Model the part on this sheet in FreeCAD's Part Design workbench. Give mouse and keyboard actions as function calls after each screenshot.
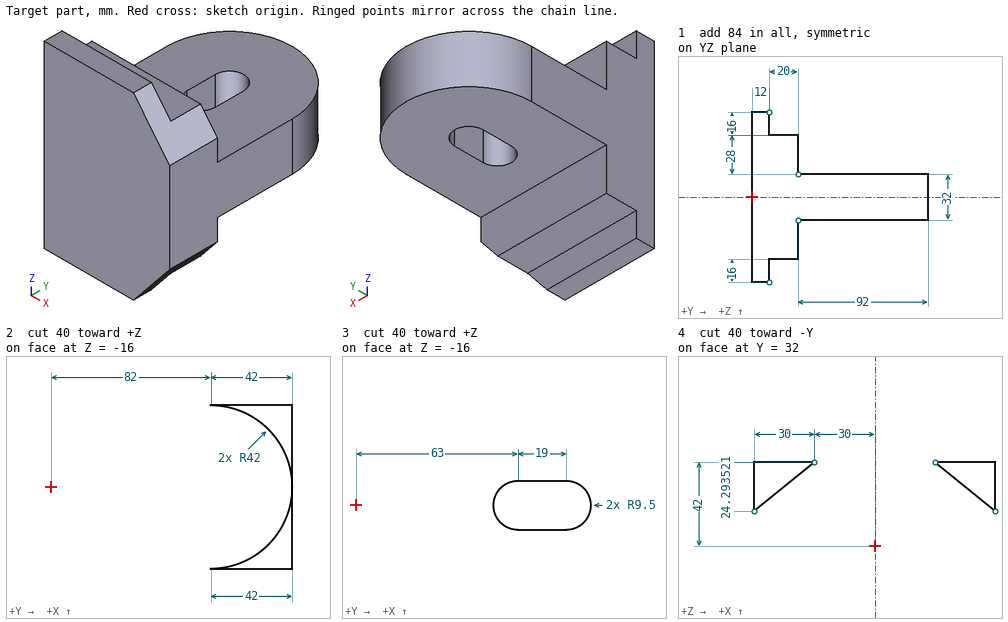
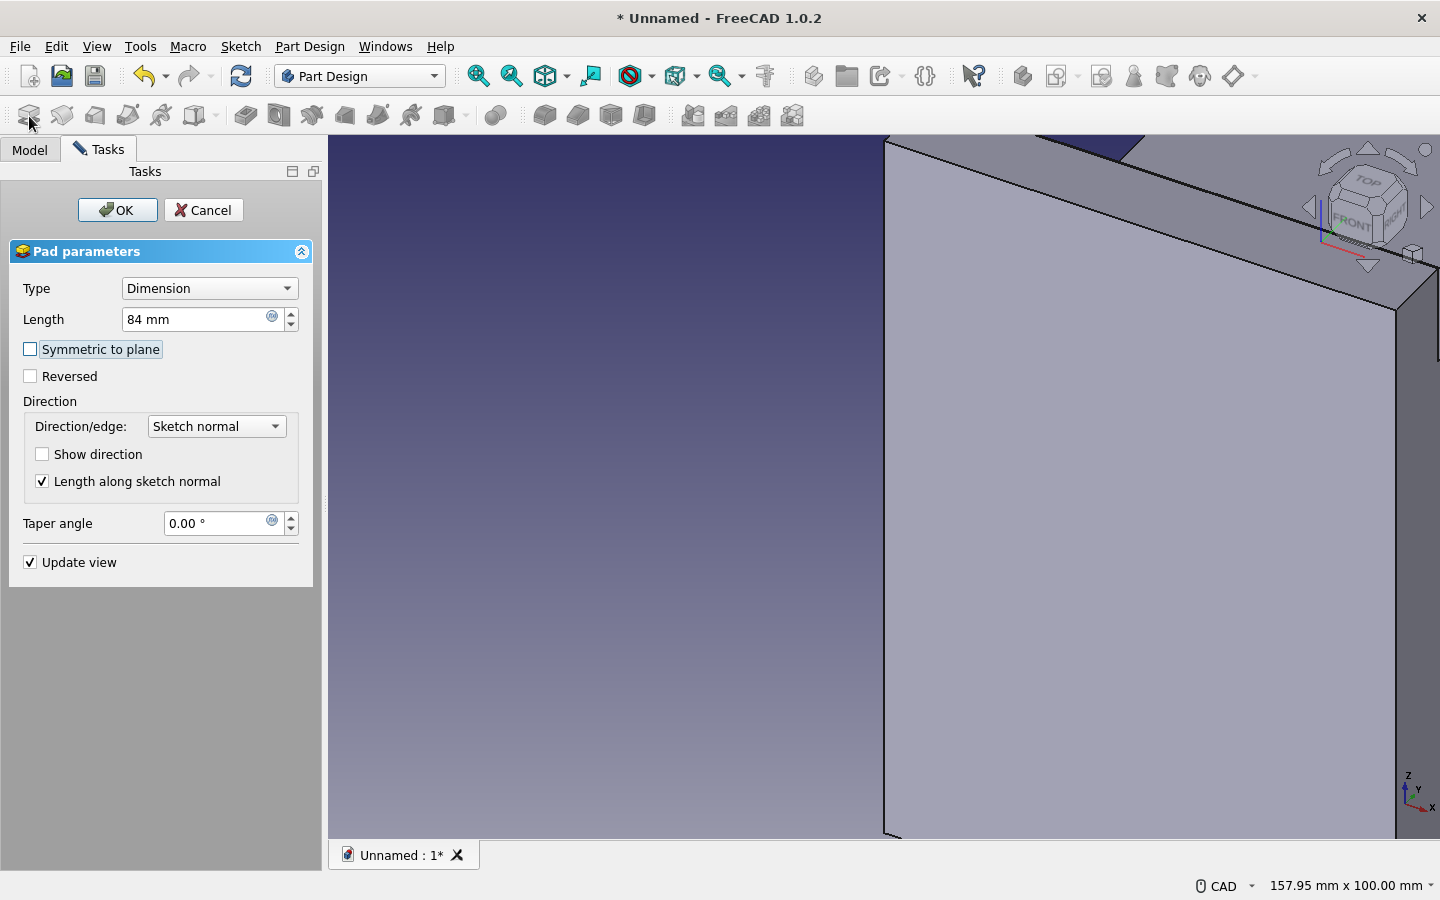
click(31, 349)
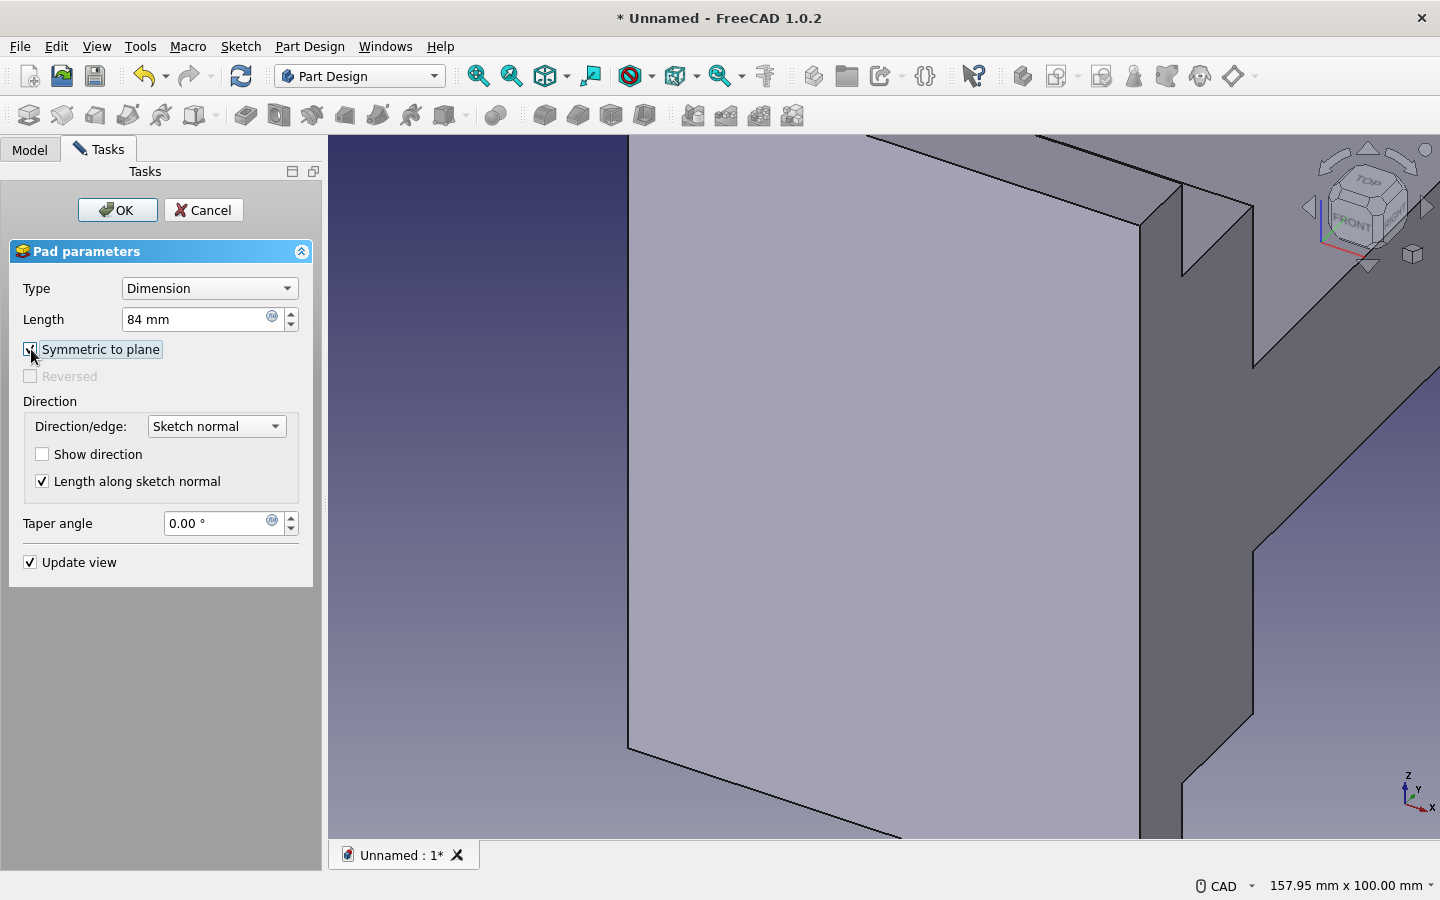
click(118, 210)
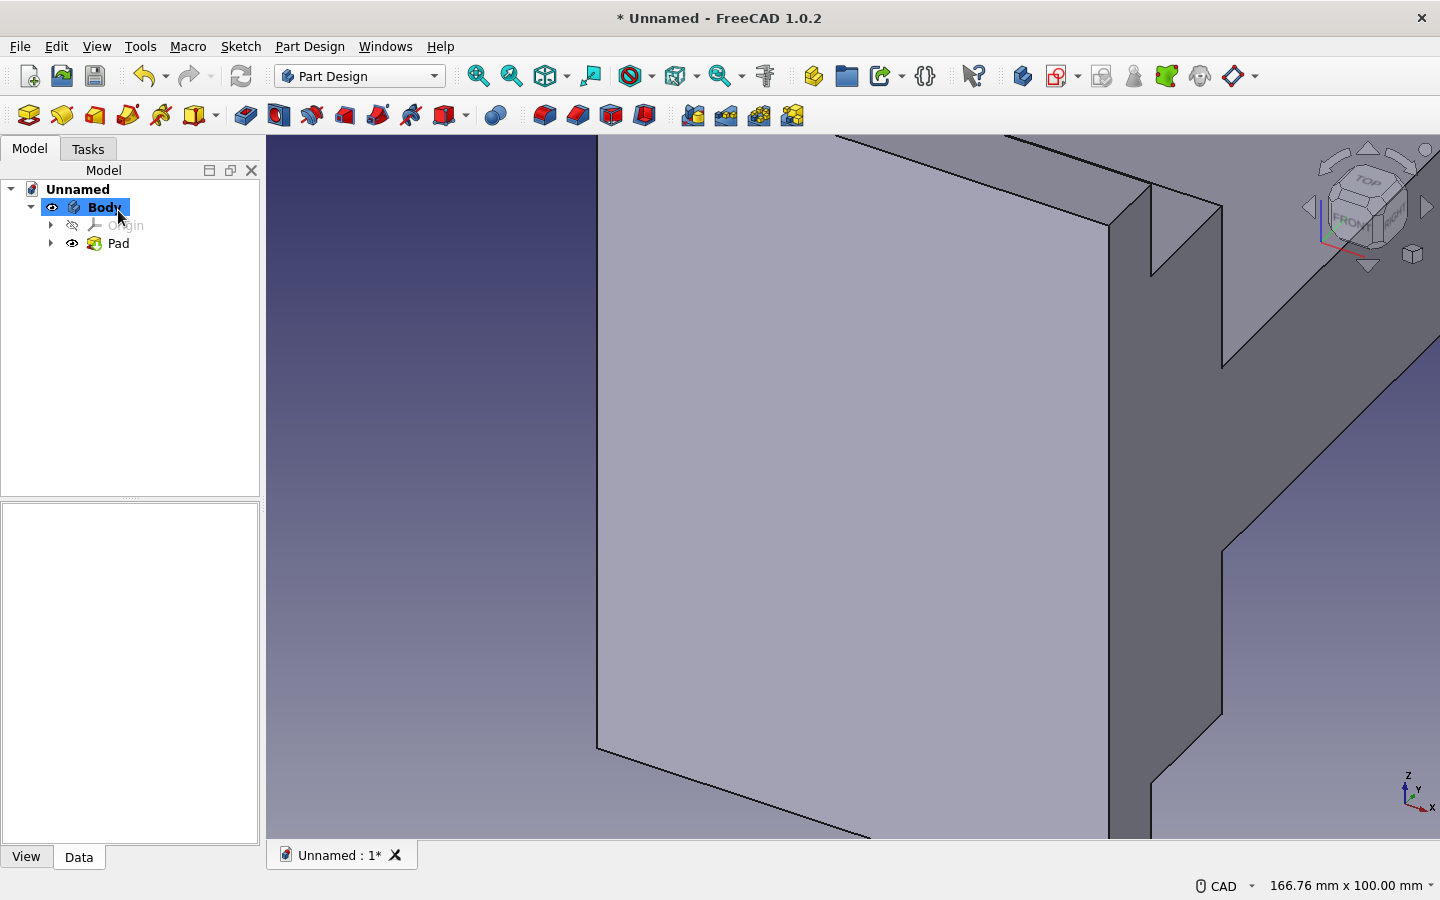
click(479, 76)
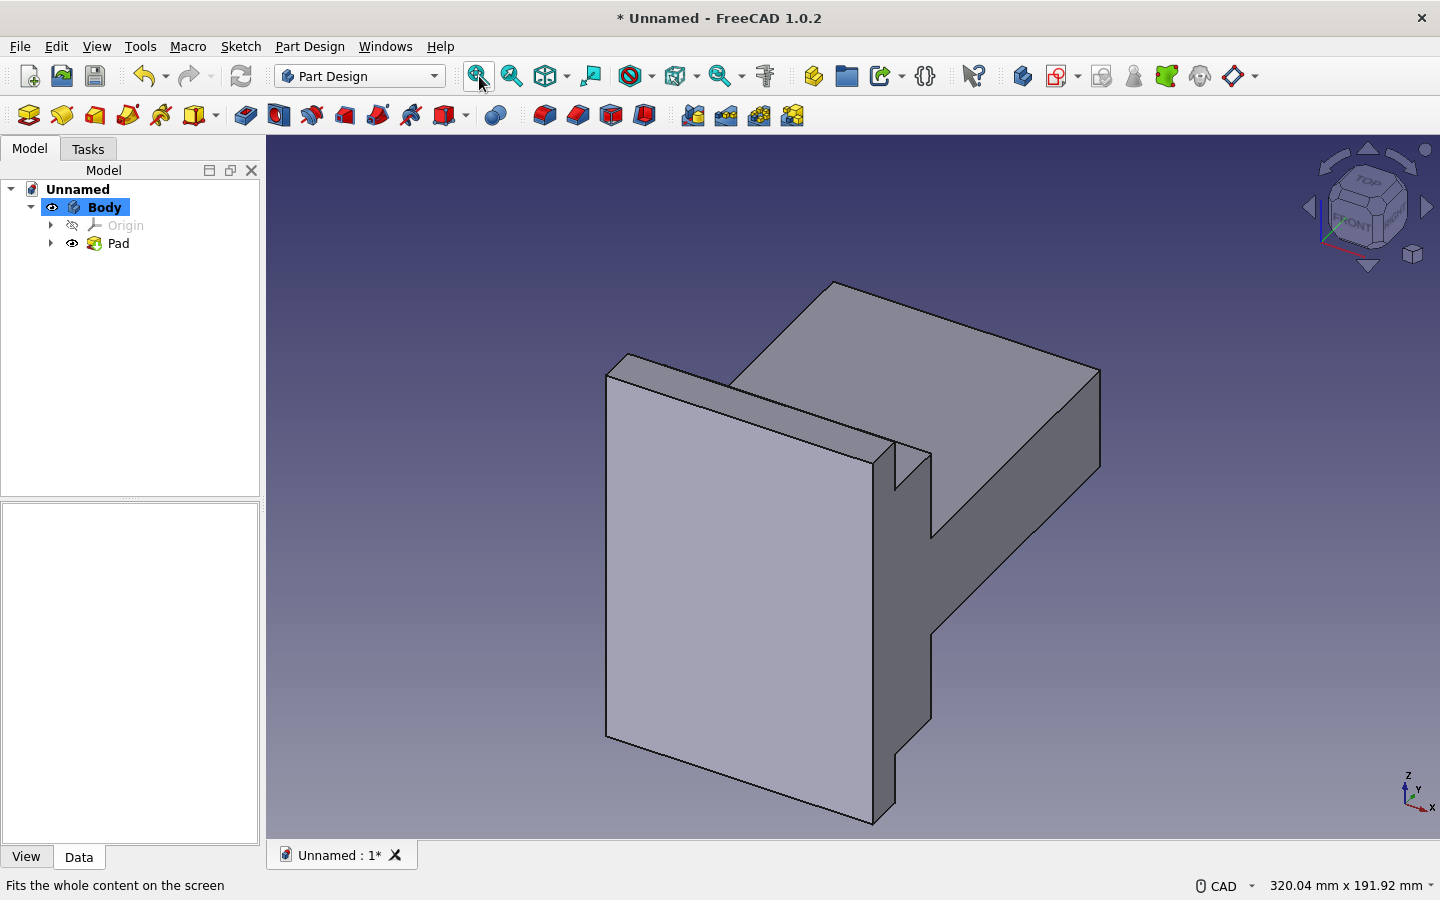
key(5)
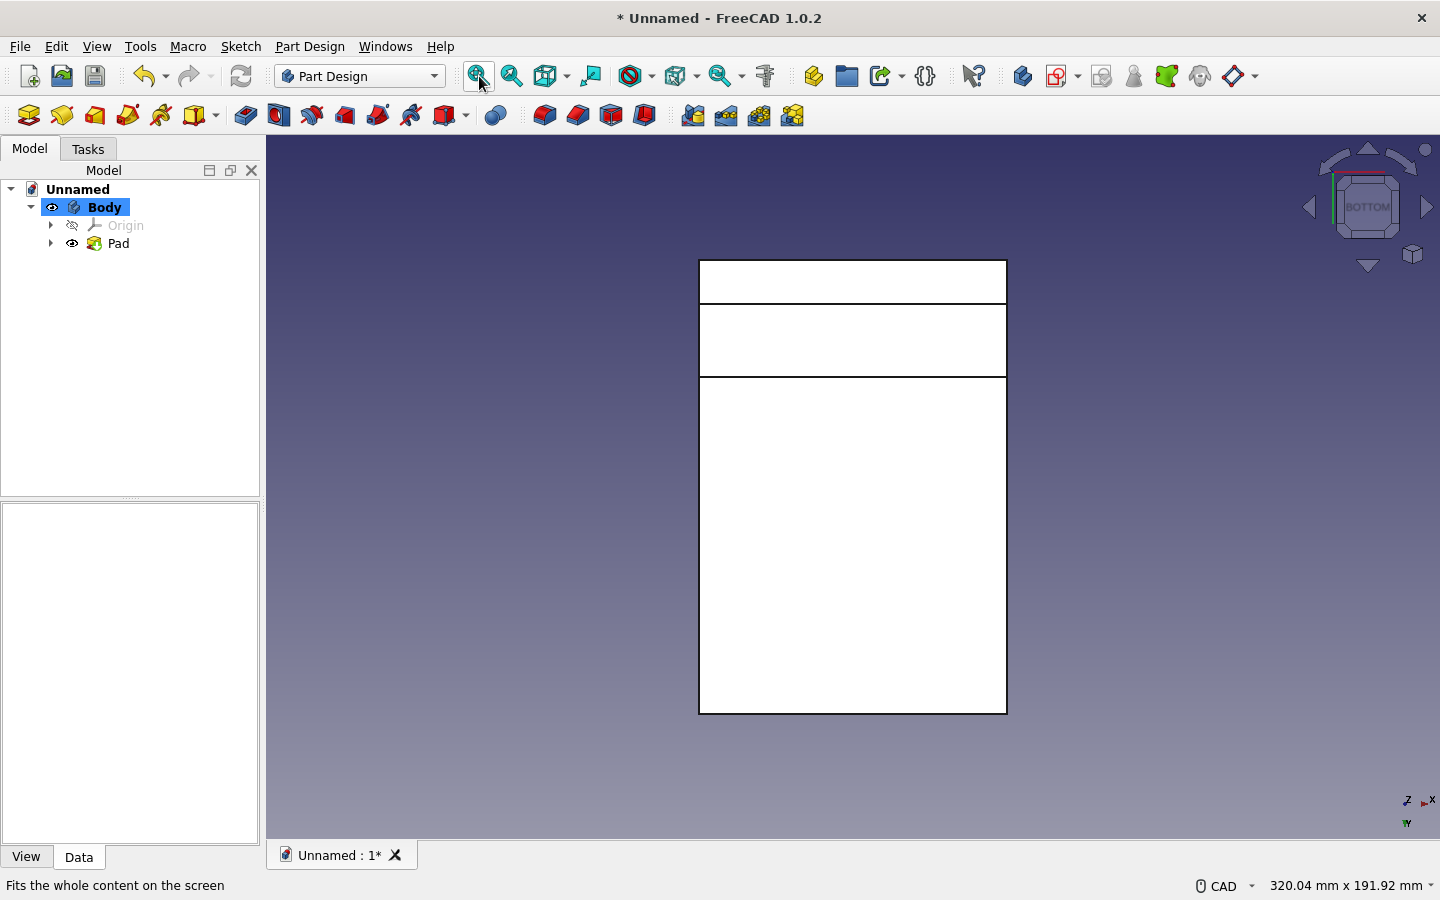
click(853, 545)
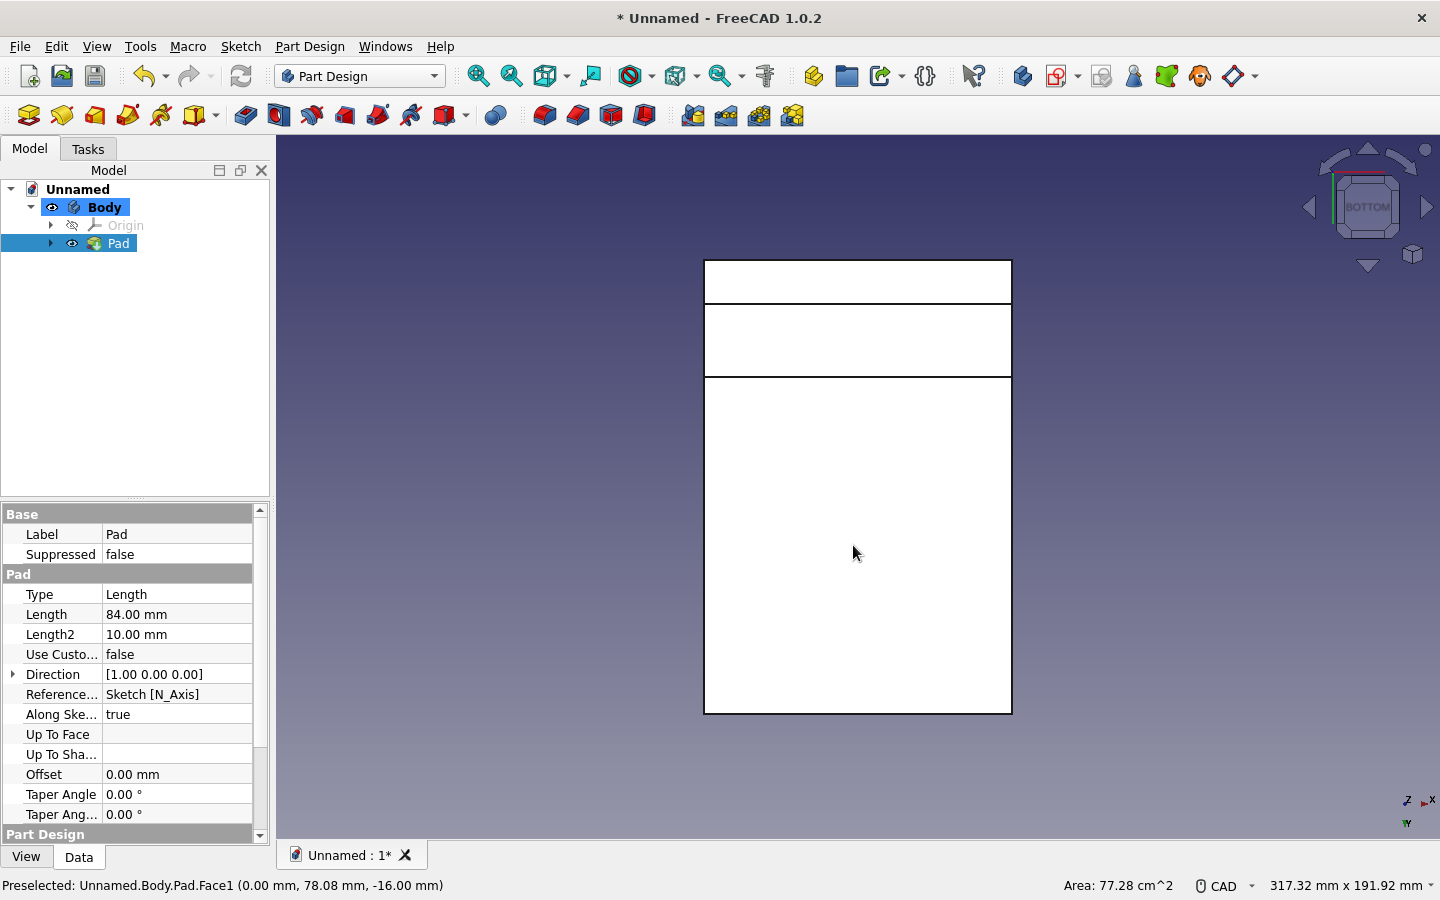
click(1056, 76)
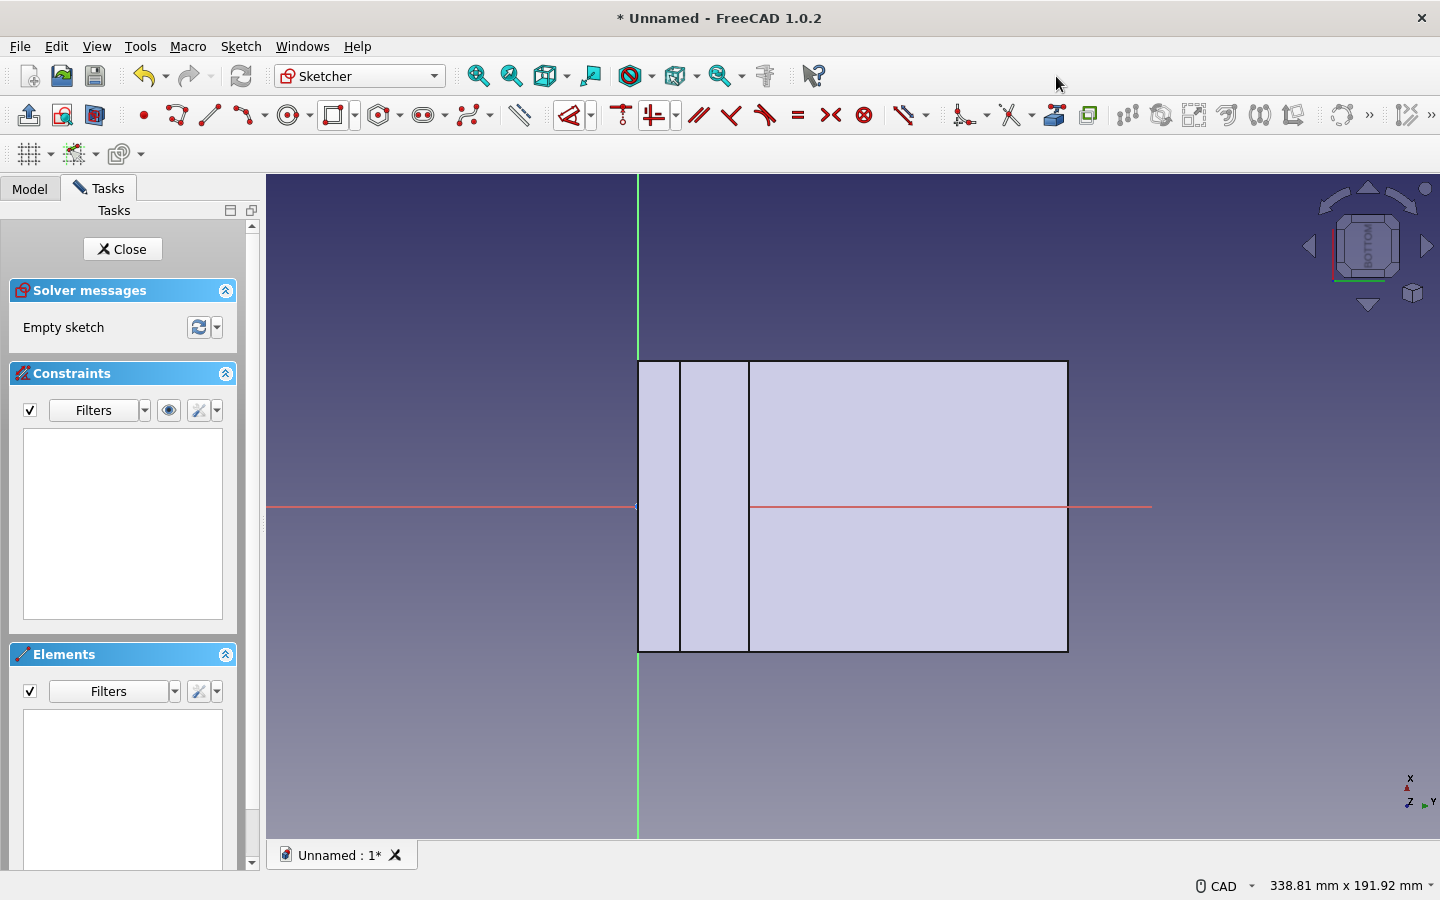
scroll(992, 506, up, 2)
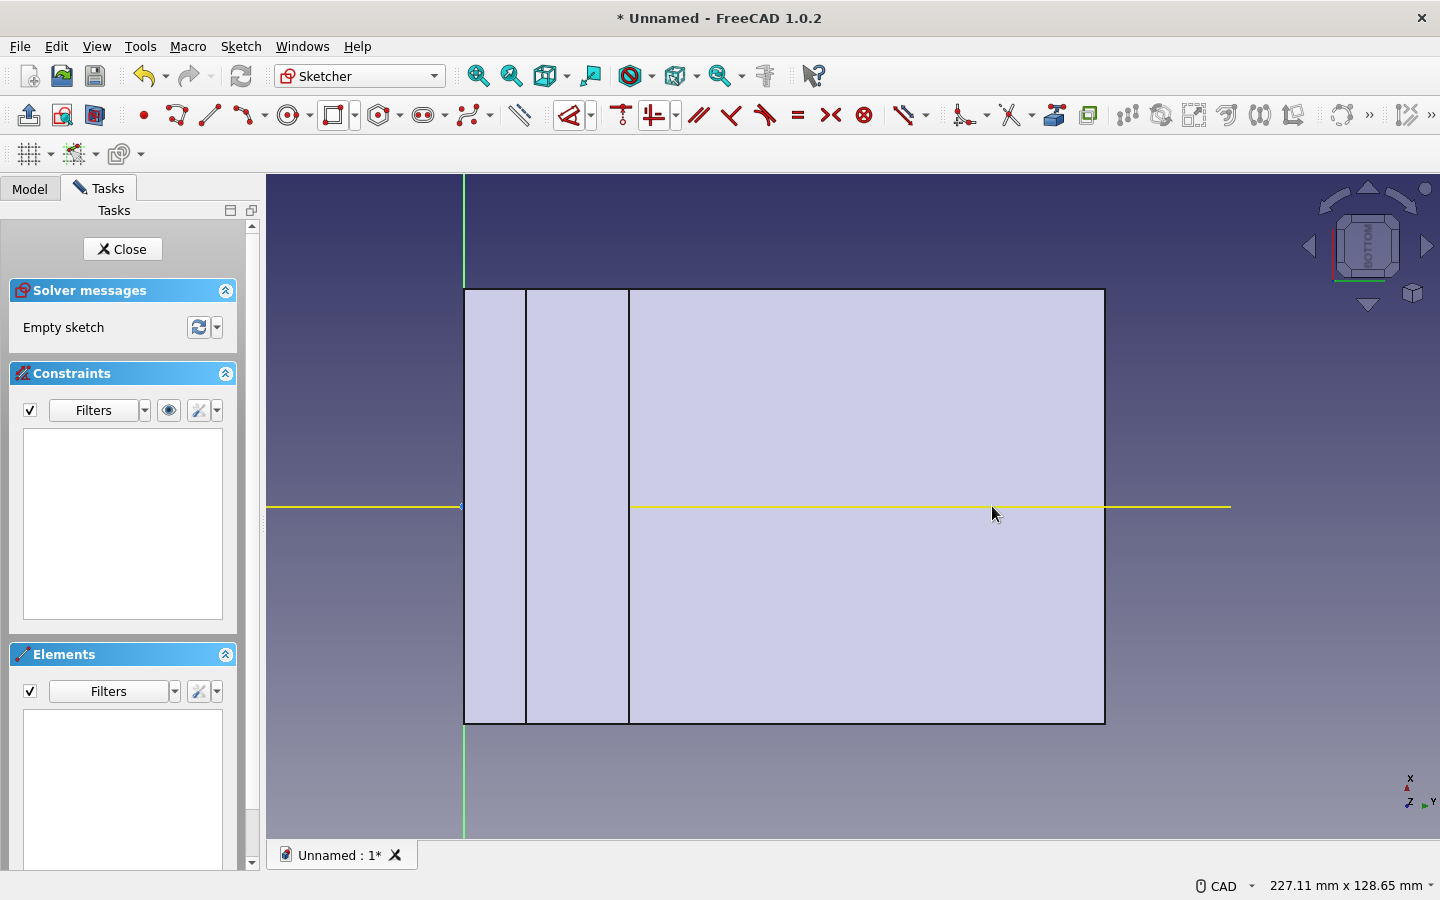
key(g)
key(m)